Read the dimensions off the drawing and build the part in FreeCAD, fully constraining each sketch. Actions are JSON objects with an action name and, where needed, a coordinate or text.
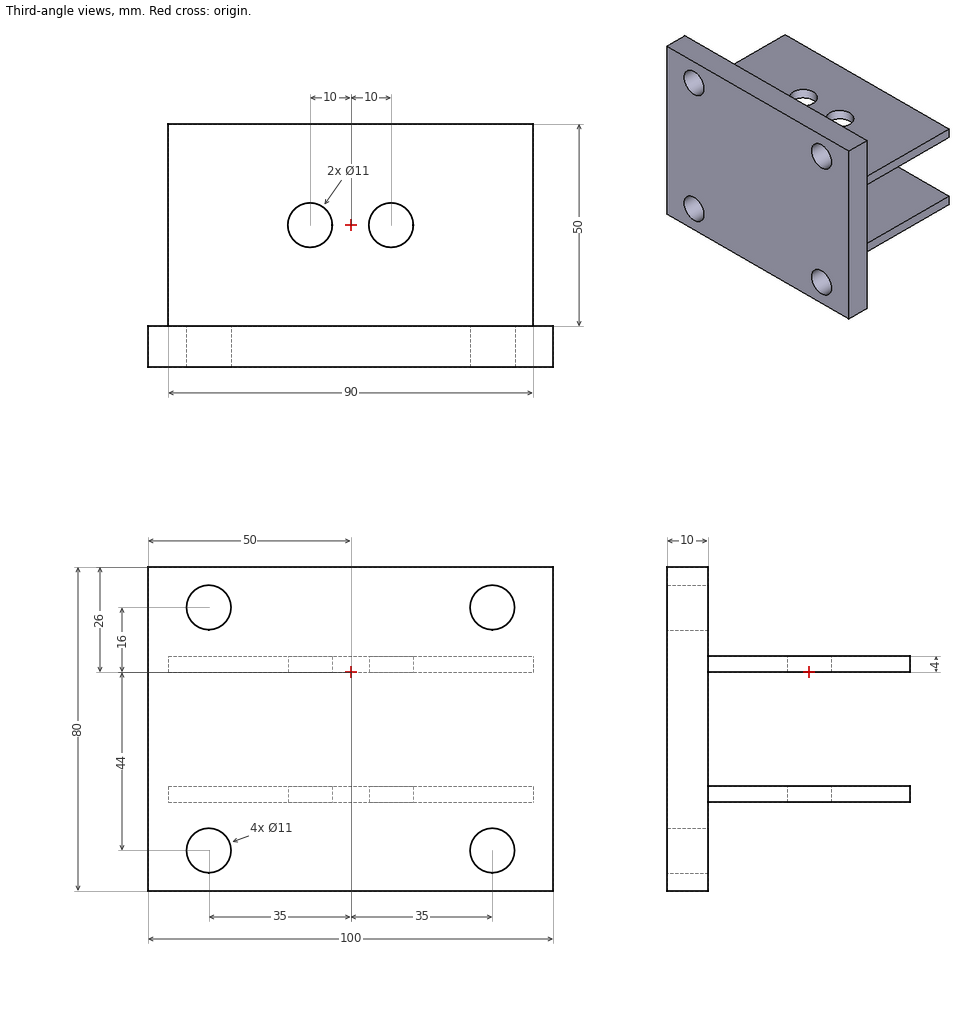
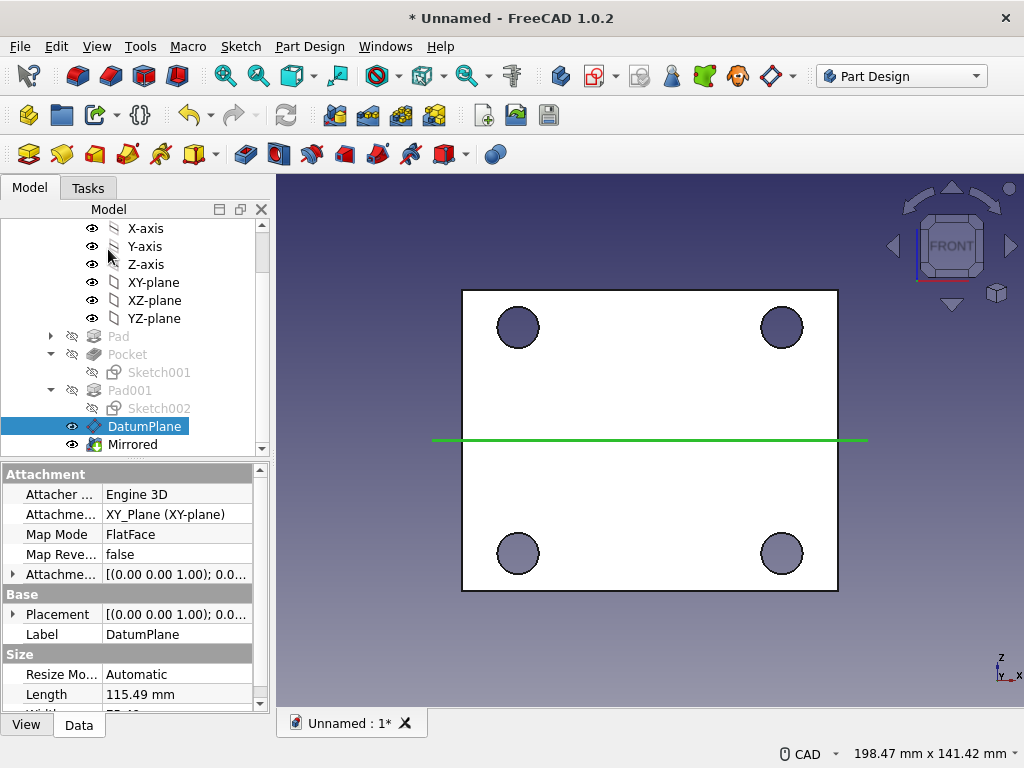
{"action": "left_click", "coordinate": [117, 426]}
{"action": "key", "text": "space"}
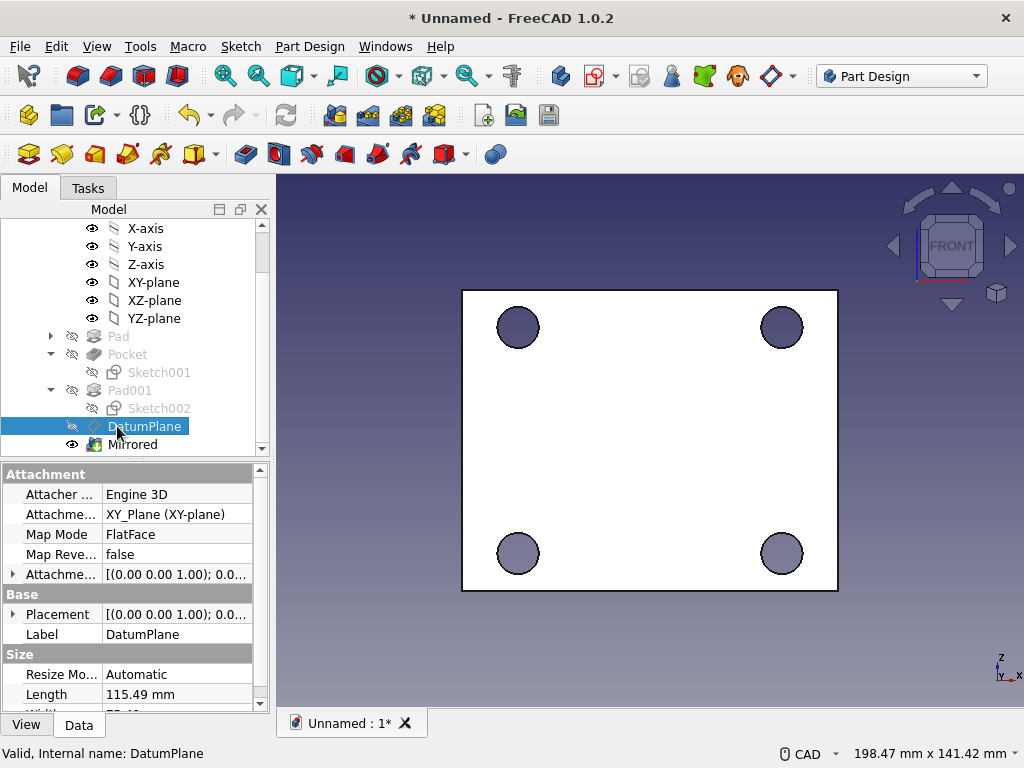
{"action": "key", "text": "0"}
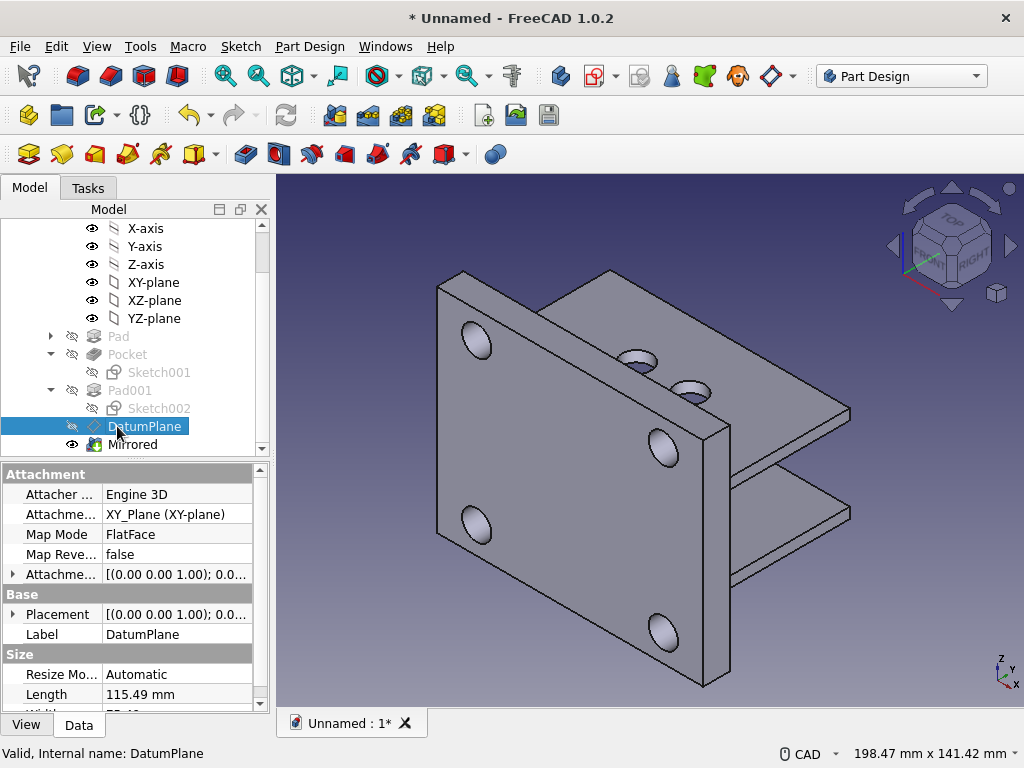
{"action": "key", "text": "2"}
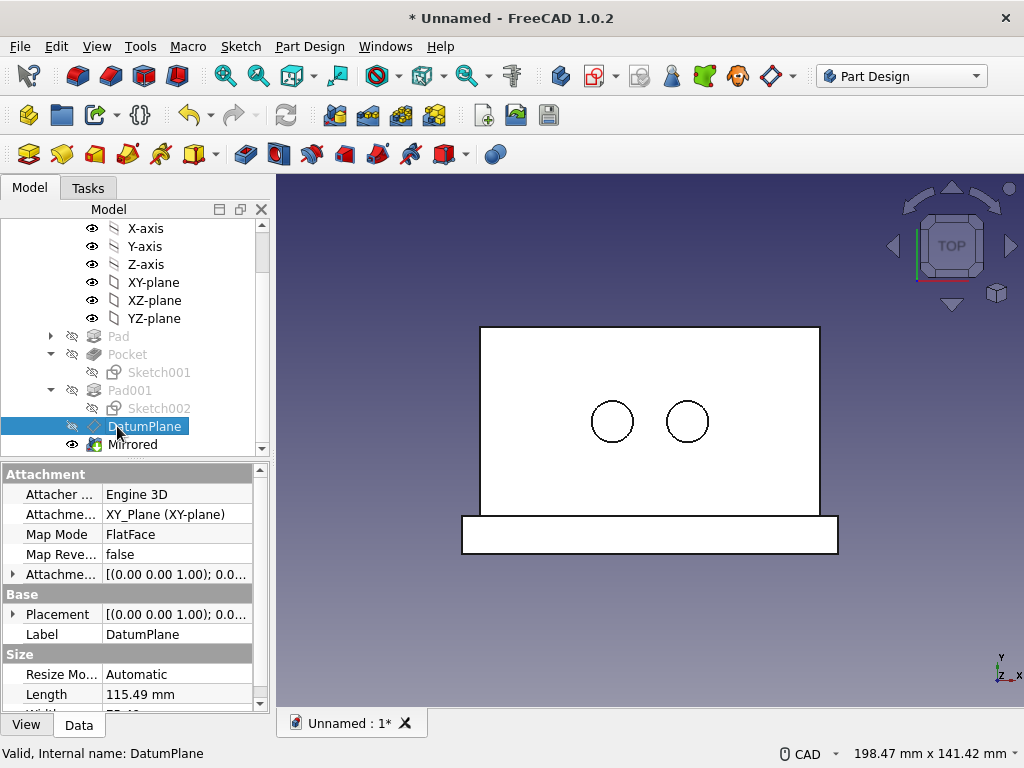
{"action": "left_click", "coordinate": [698, 421]}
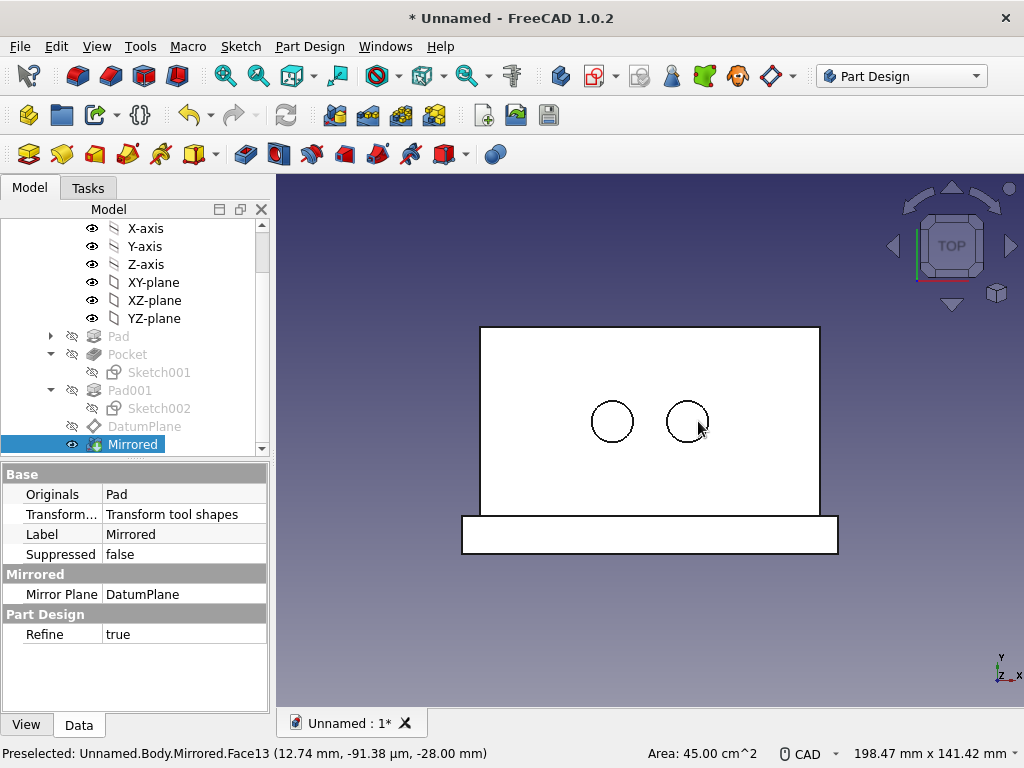
{"action": "left_click", "coordinate": [594, 76]}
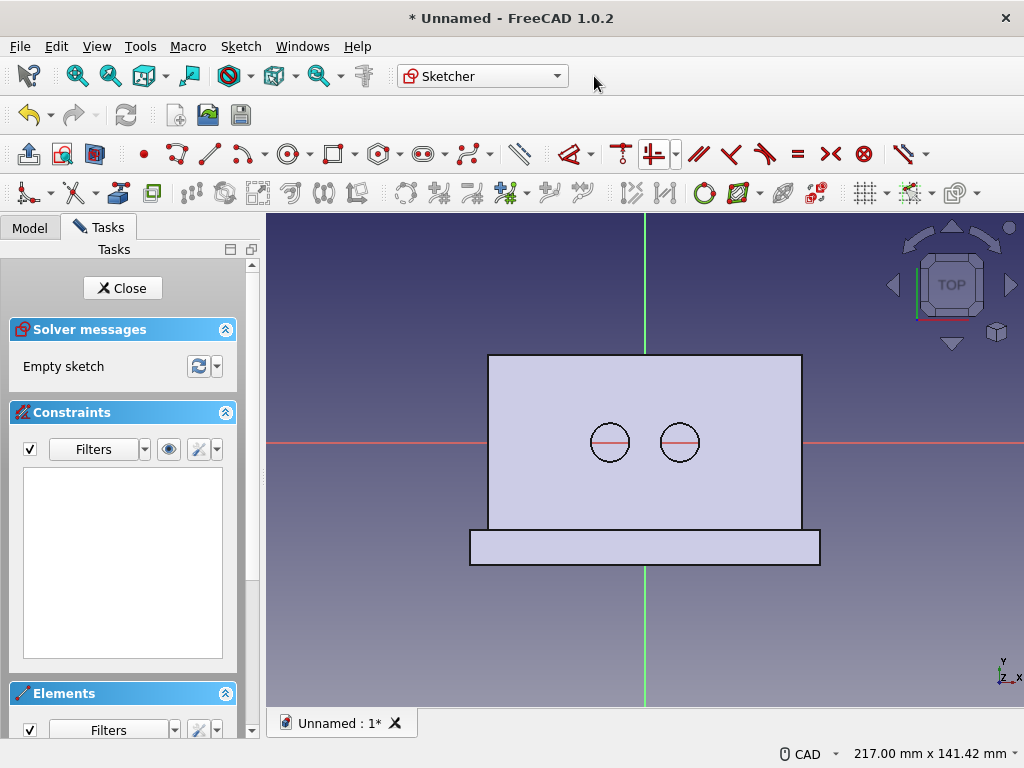
{"action": "key", "text": "q s"}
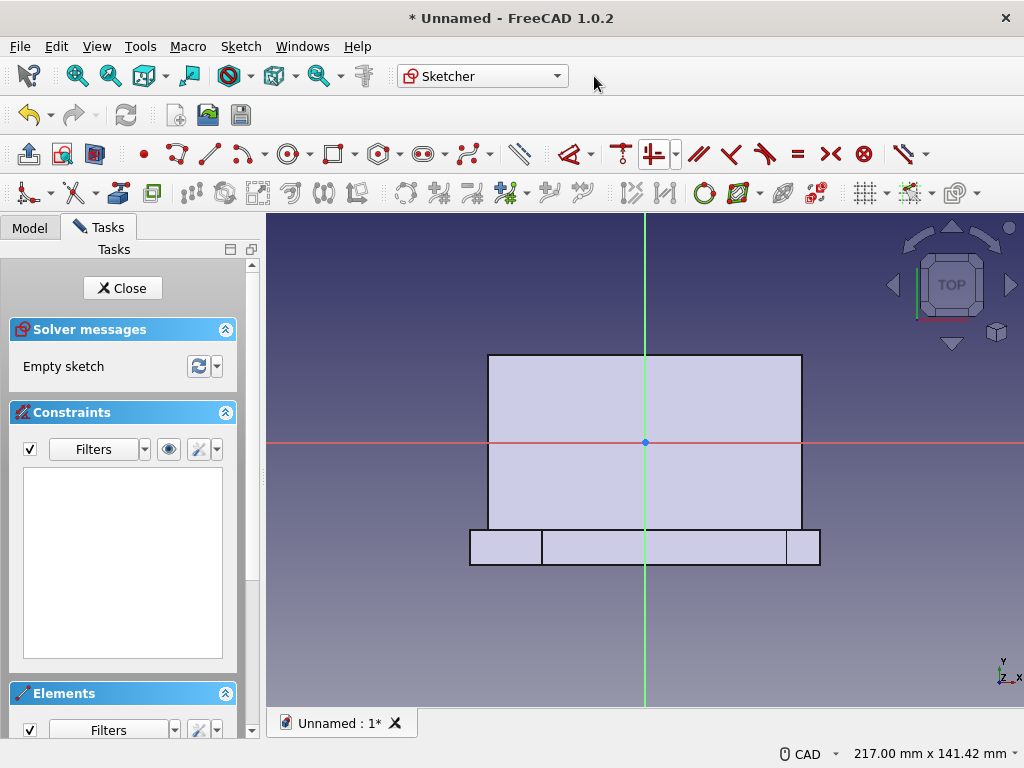
{"action": "scroll", "coordinate": [667, 437], "scroll_direction": "up", "scroll_amount": 7}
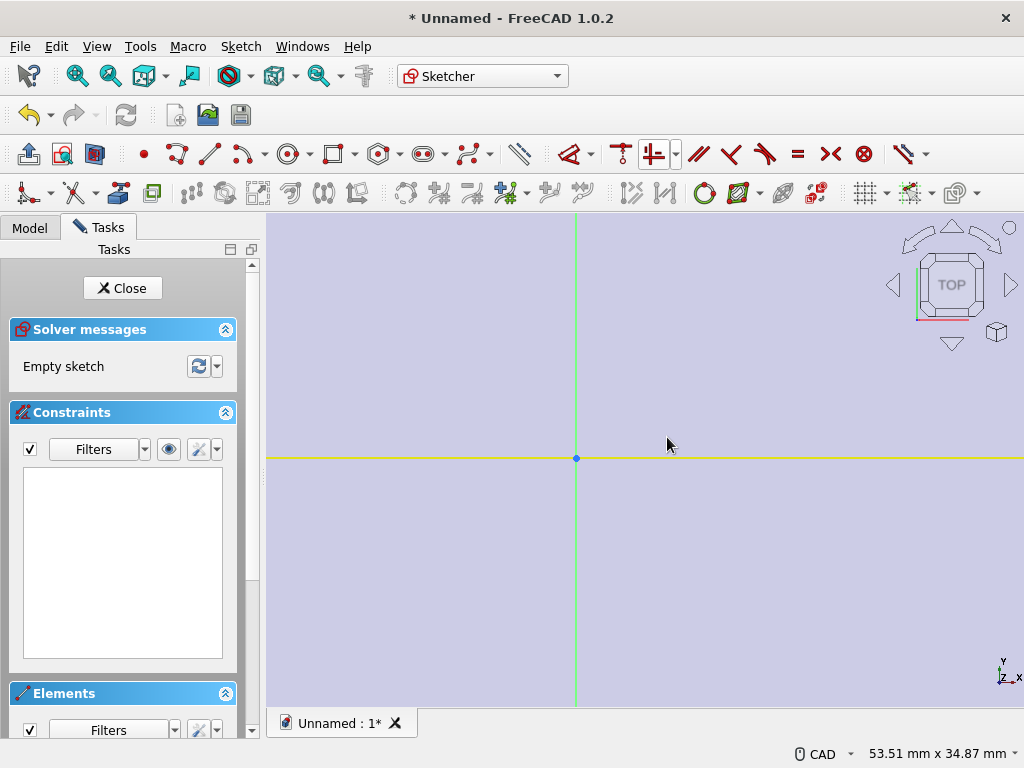
{"action": "key", "text": "g c"}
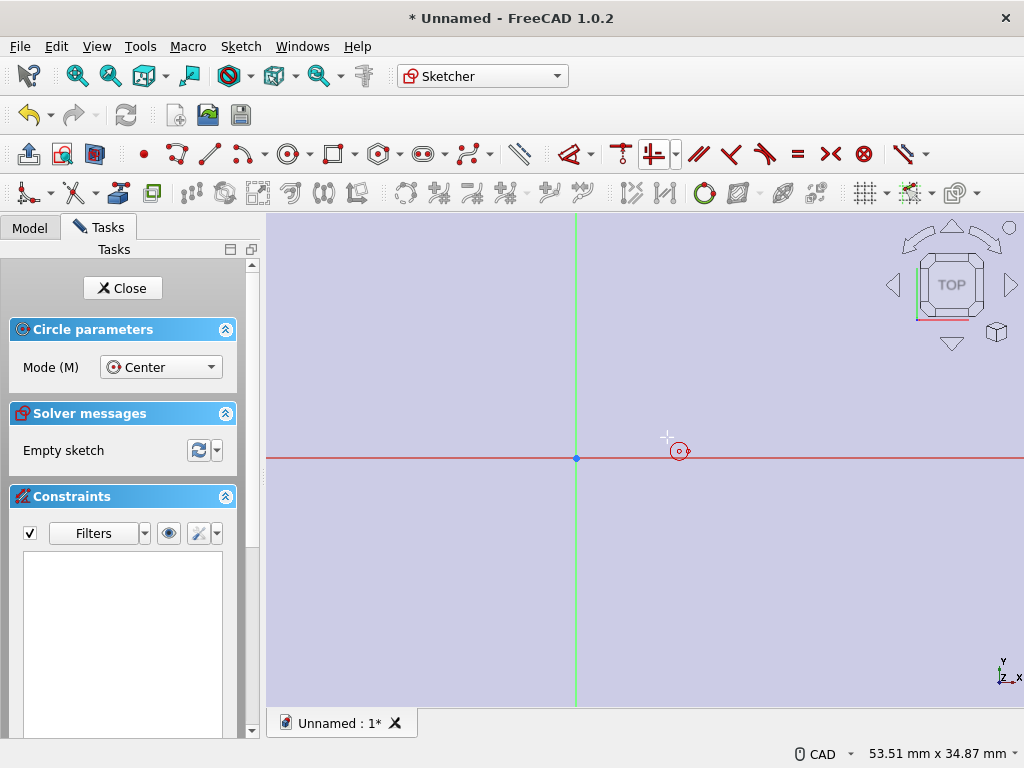
{"action": "left_click", "coordinate": [435, 458]}
{"action": "left_click", "coordinate": [490, 403]}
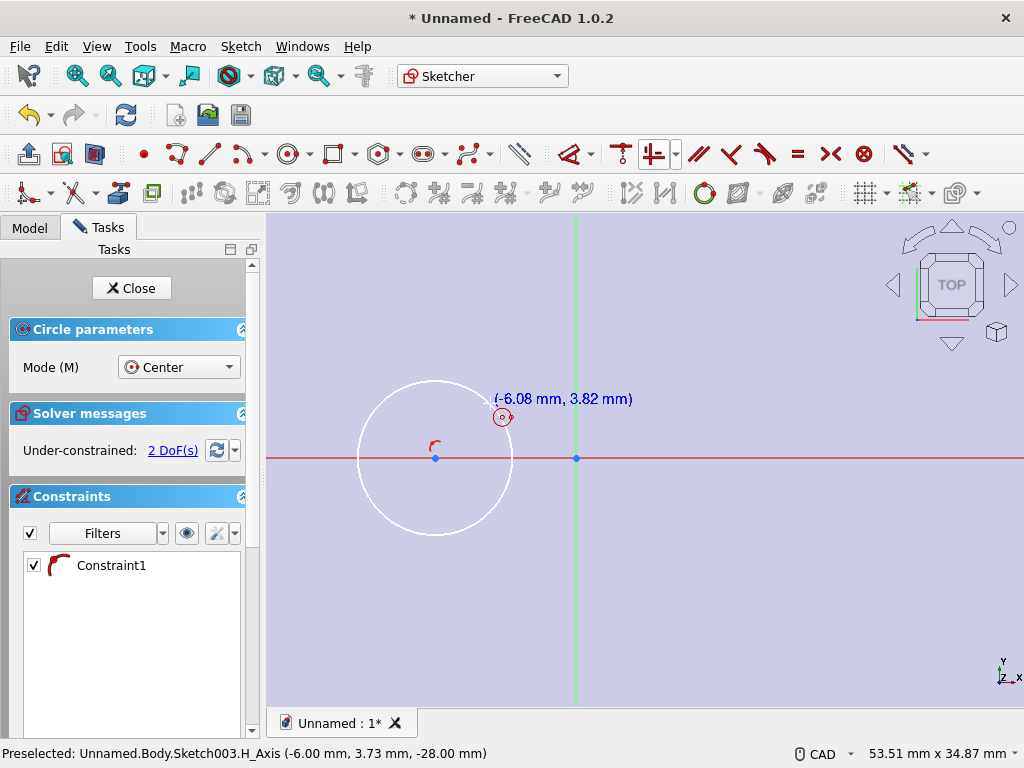
{"action": "left_click", "coordinate": [718, 458]}
{"action": "left_click", "coordinate": [773, 403]}
{"action": "key", "text": "Escape"}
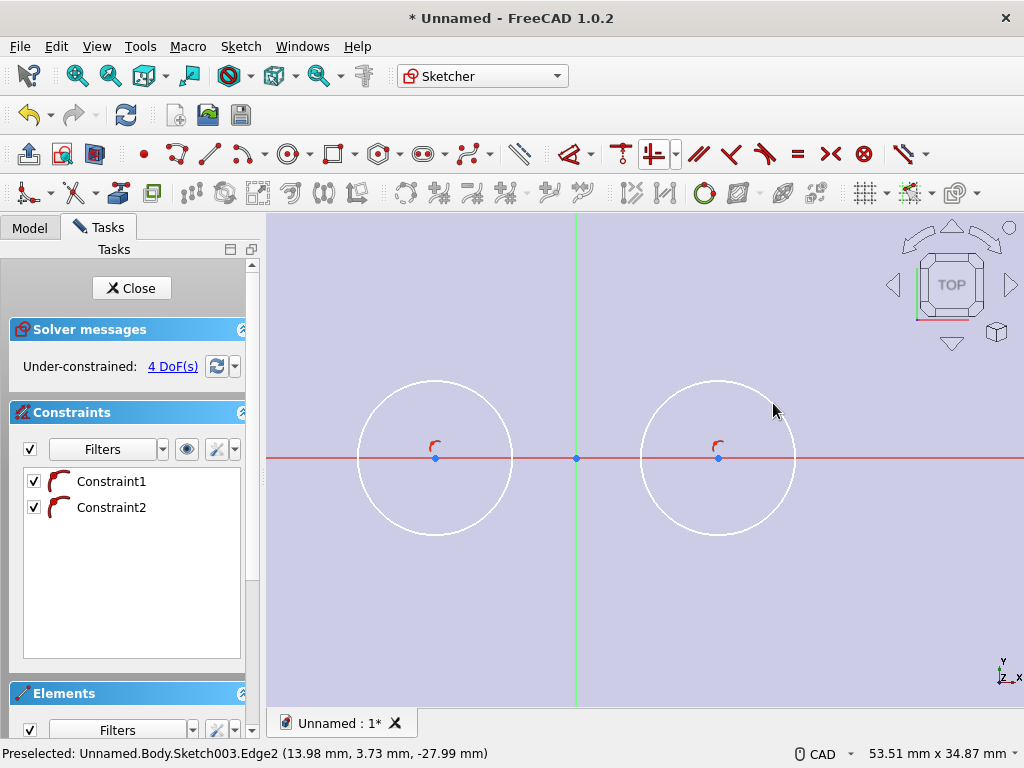
{"action": "left_click", "coordinate": [489, 403]}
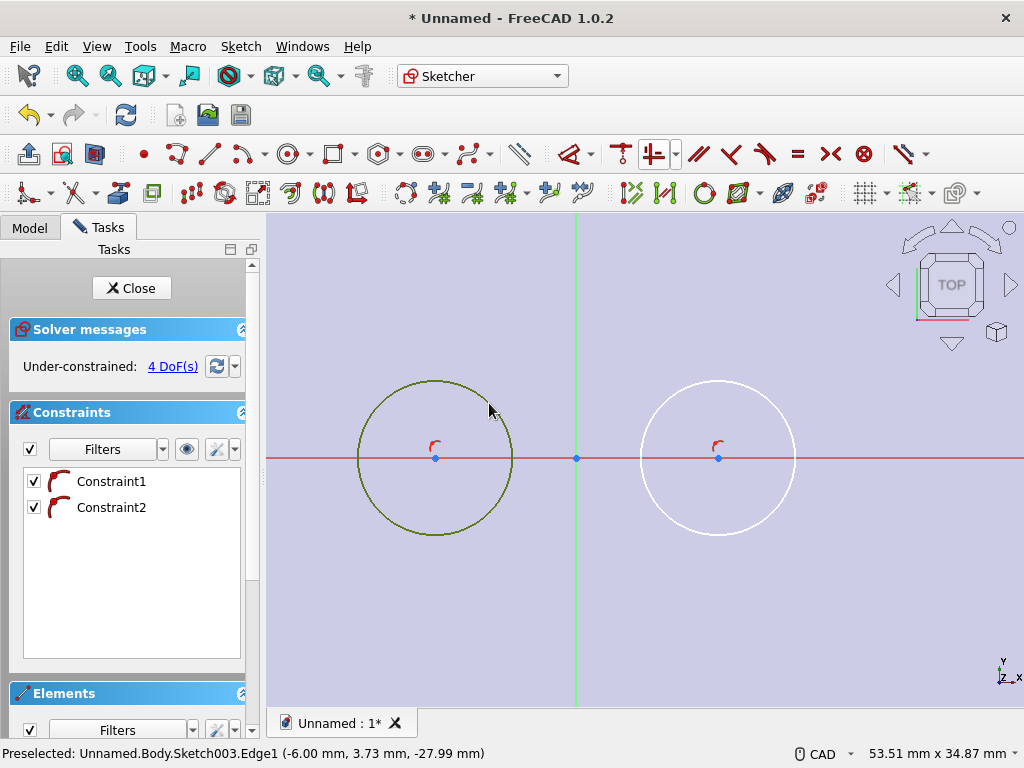
{"action": "left_click", "coordinate": [772, 403]}